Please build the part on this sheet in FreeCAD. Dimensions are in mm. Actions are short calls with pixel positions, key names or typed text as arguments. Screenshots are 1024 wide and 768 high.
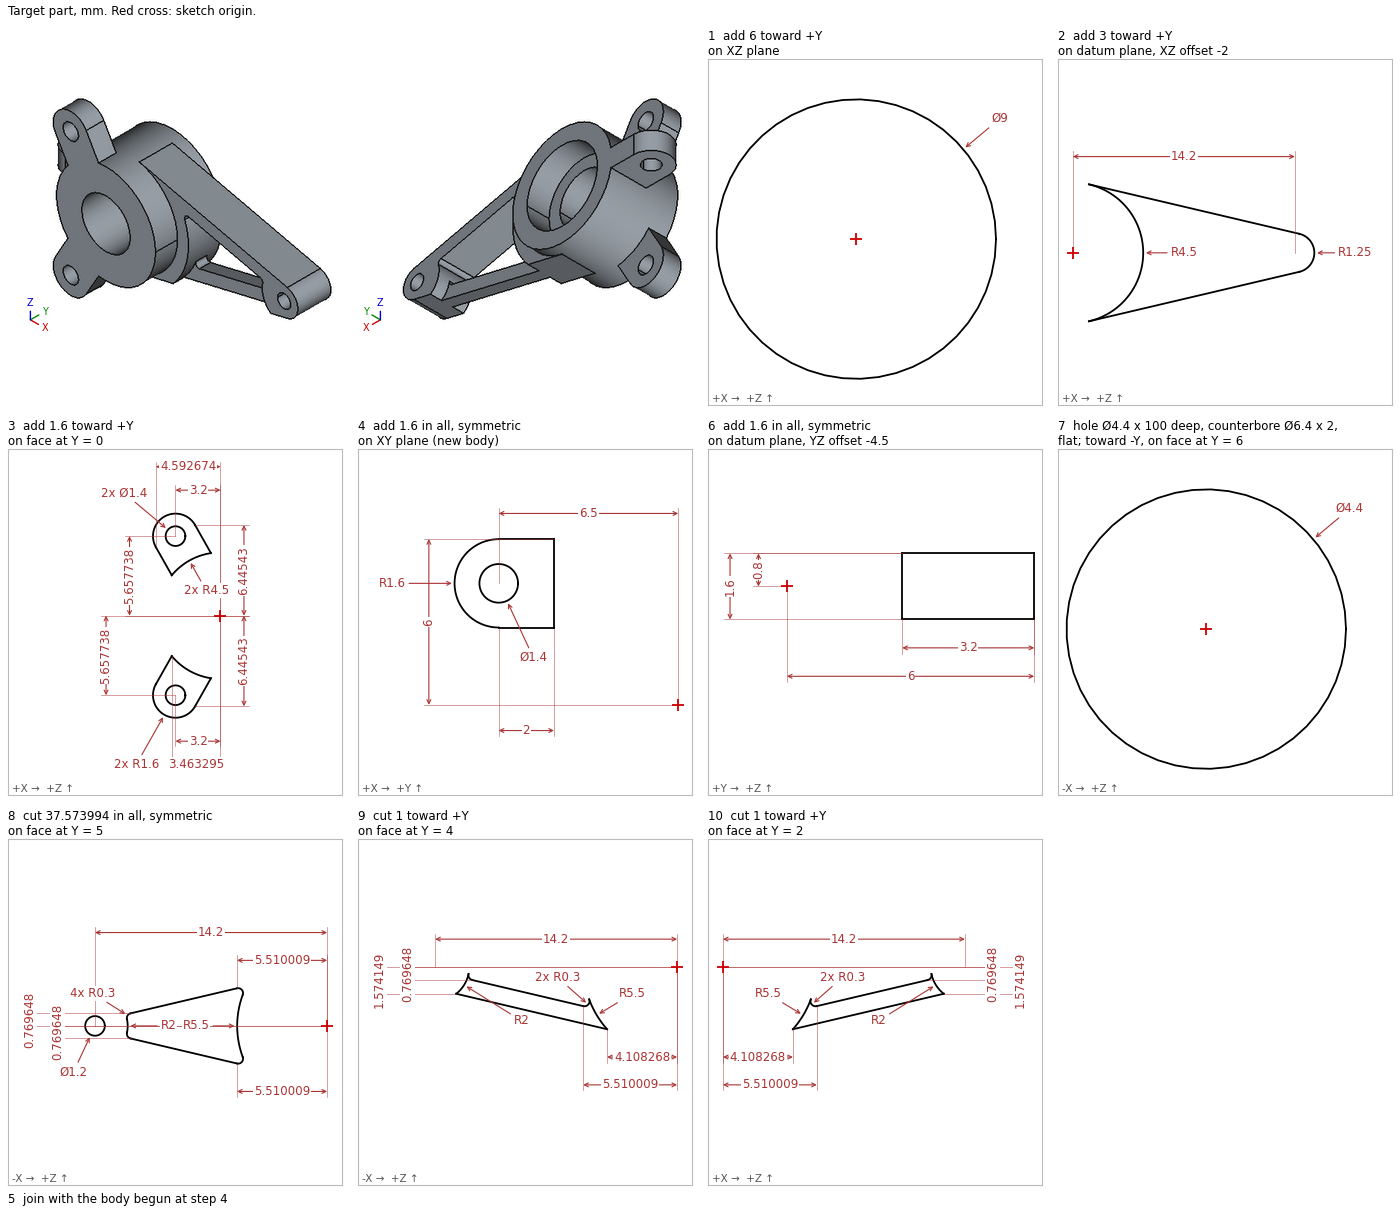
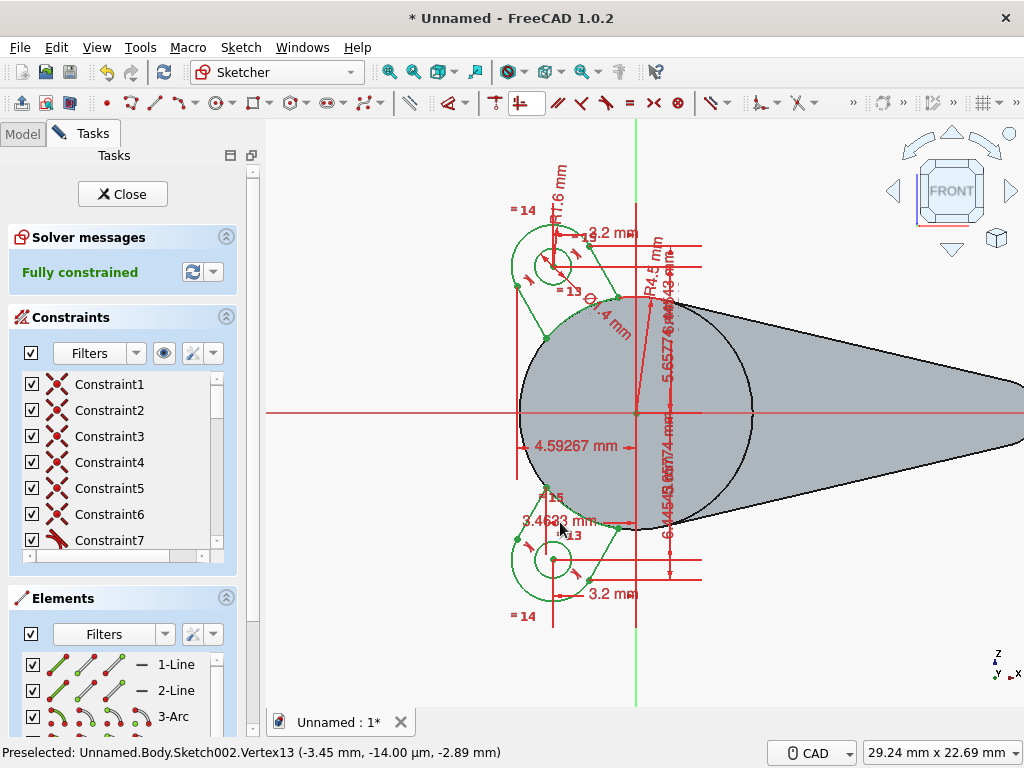
click(123, 194)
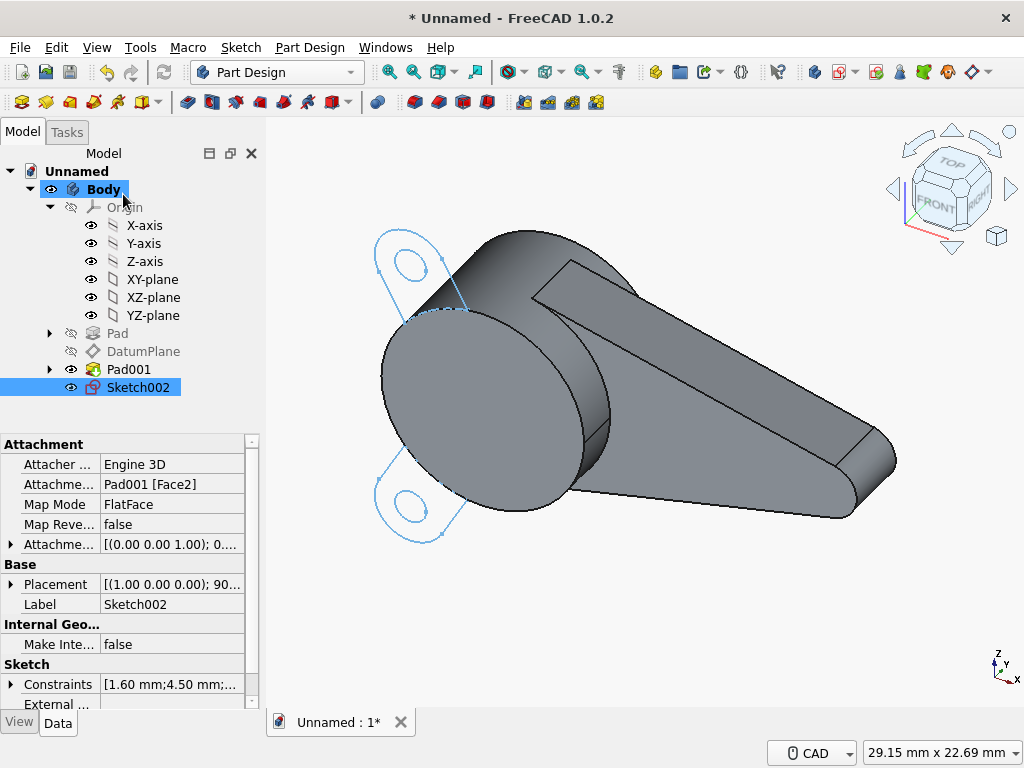
click(22, 102)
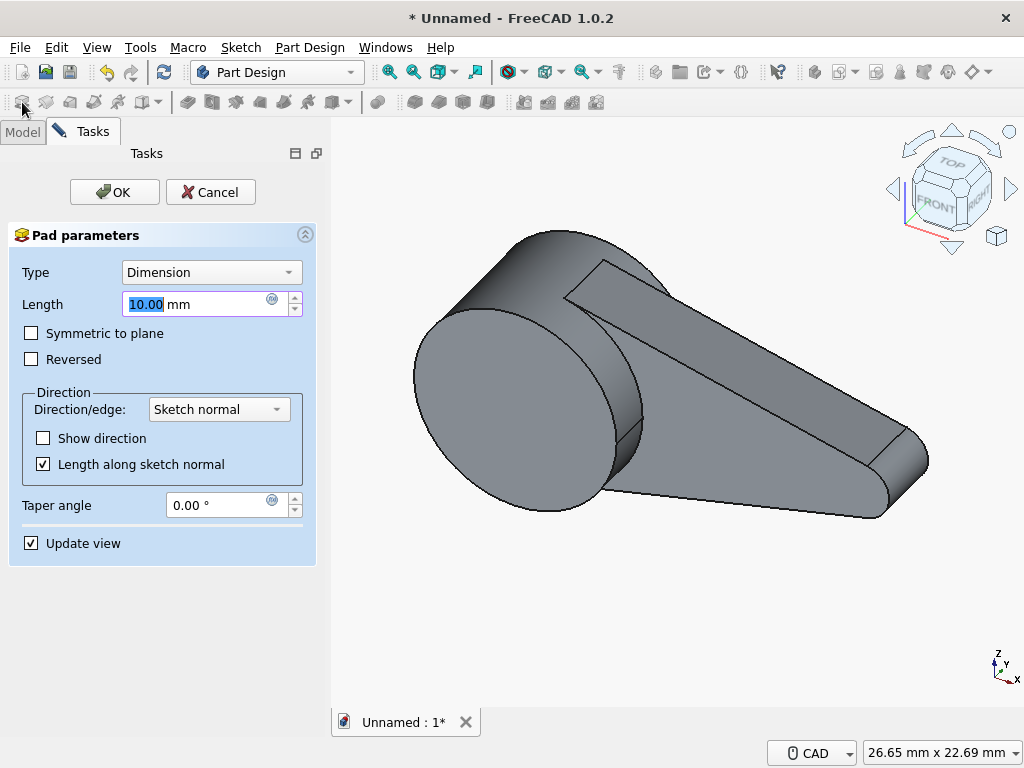
text(1.6)
key(Tab)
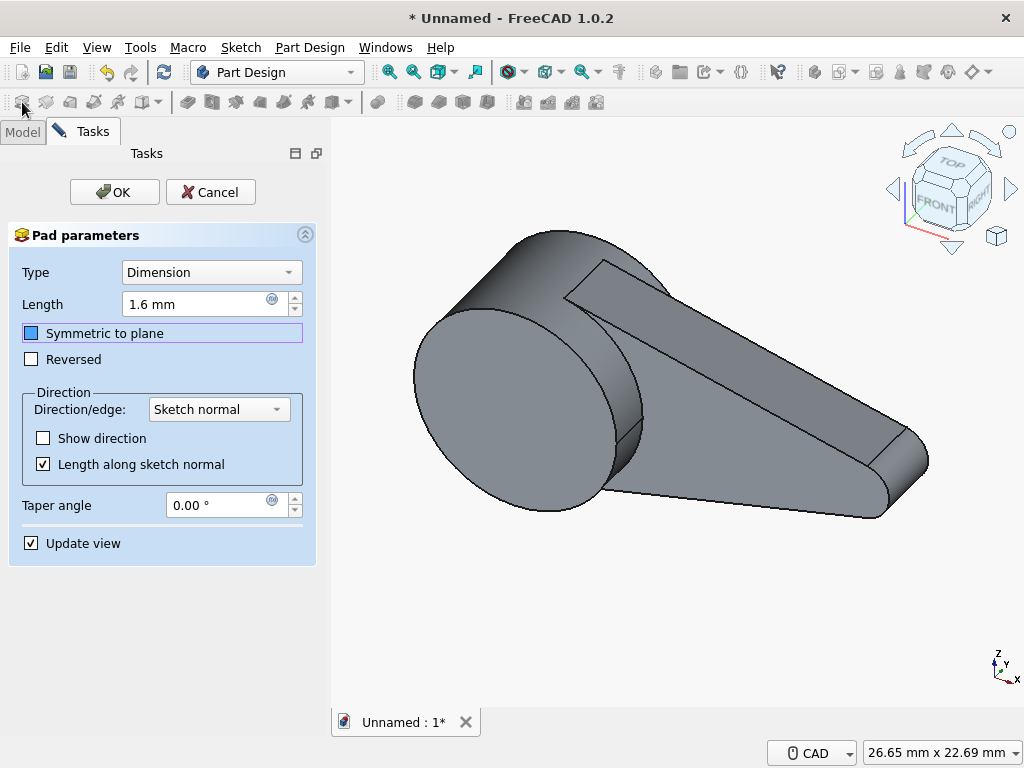
click(30, 359)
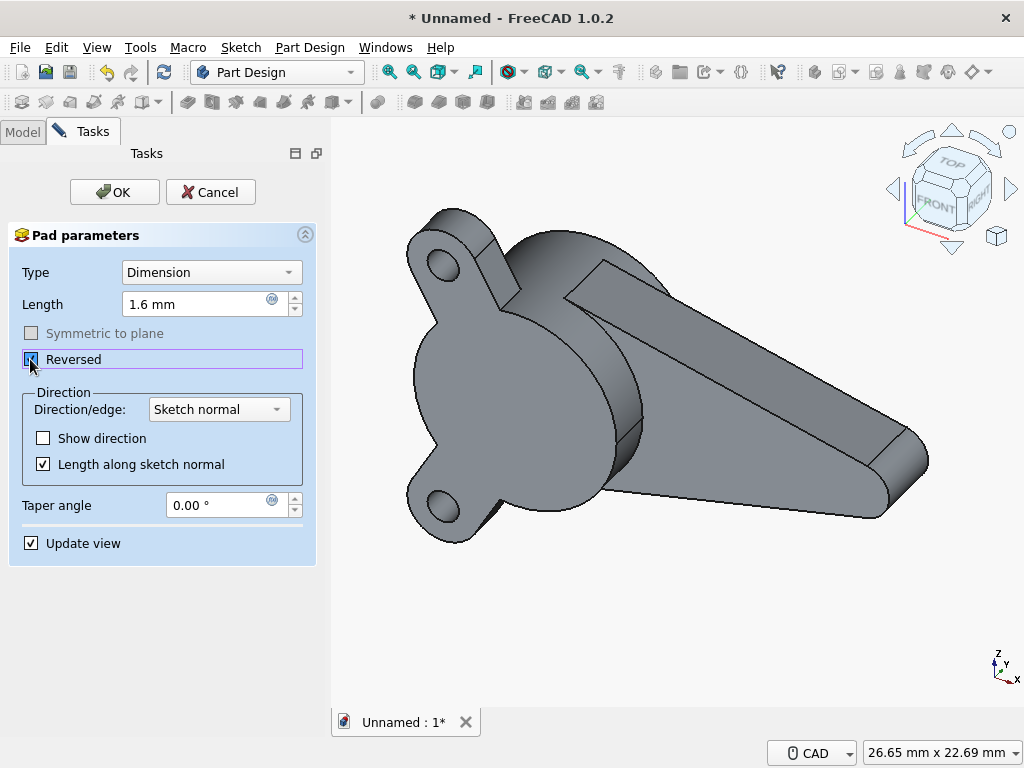
click(115, 192)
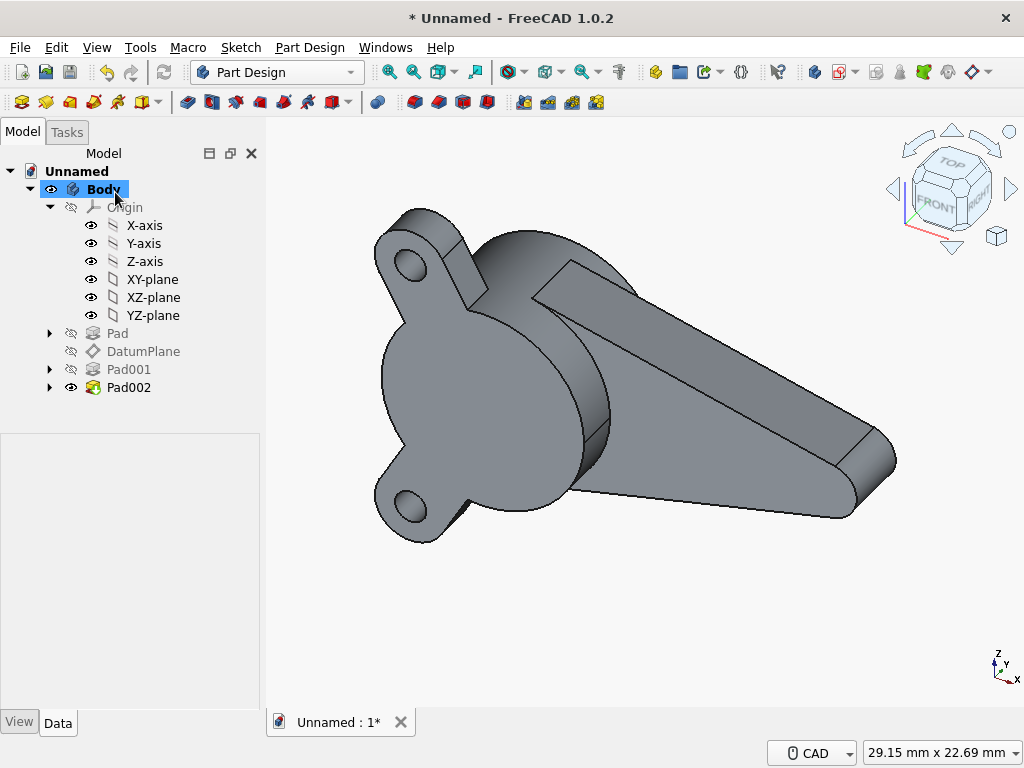
click(816, 72)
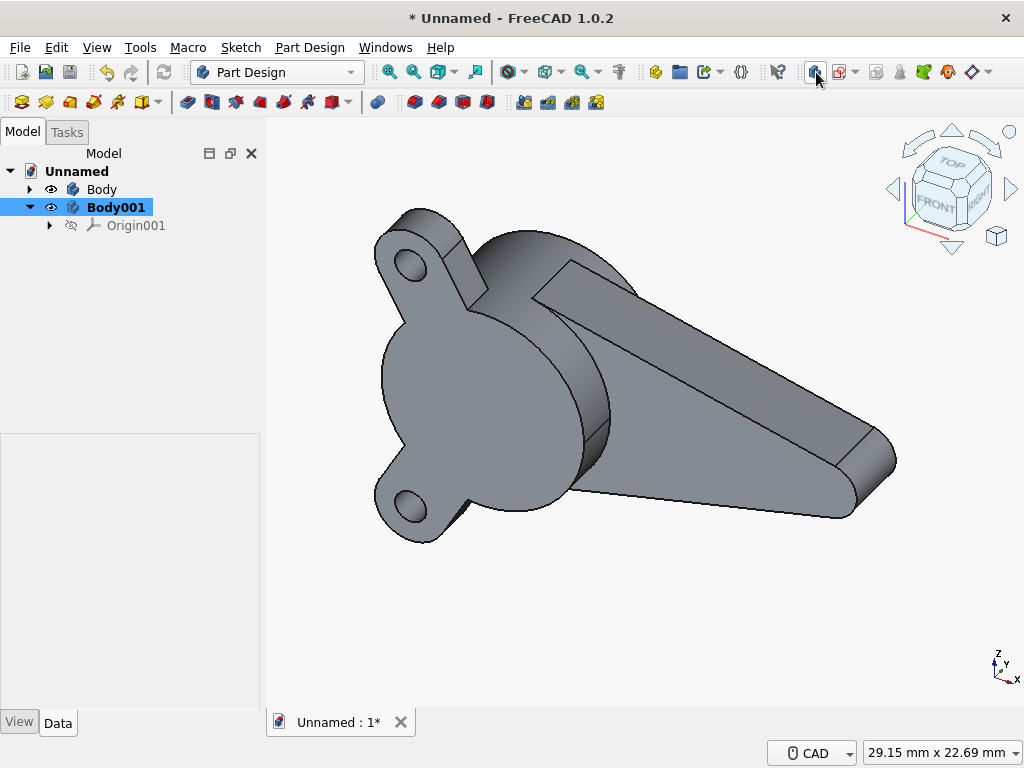
click(306, 667)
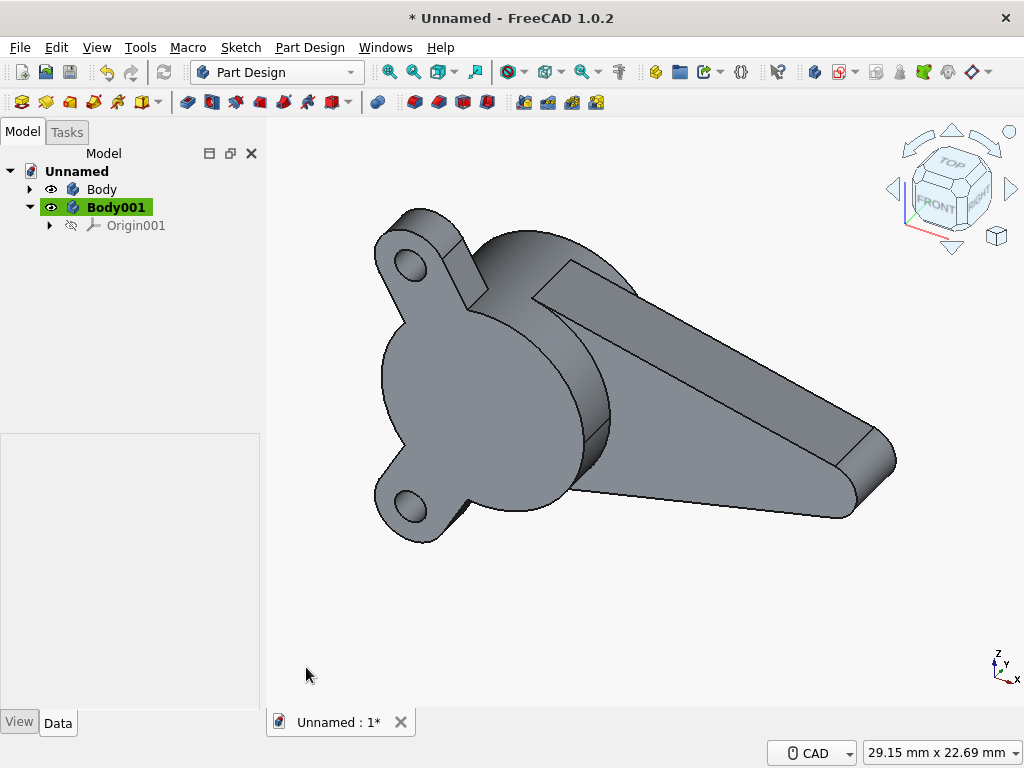
click(840, 72)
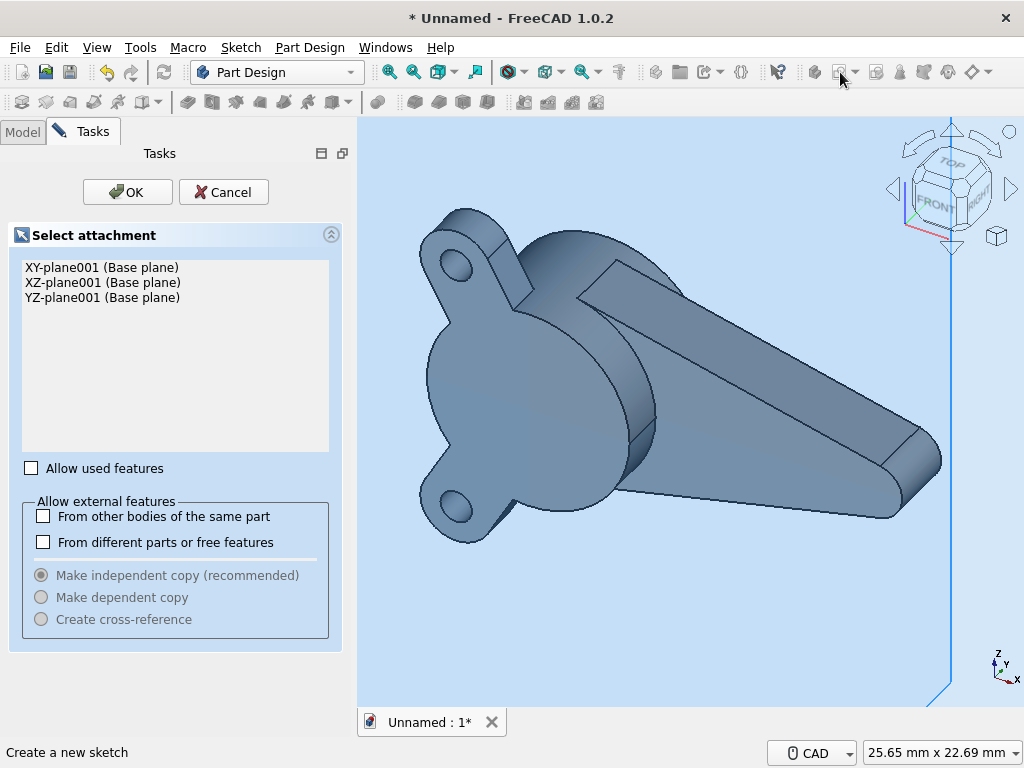
click(82, 268)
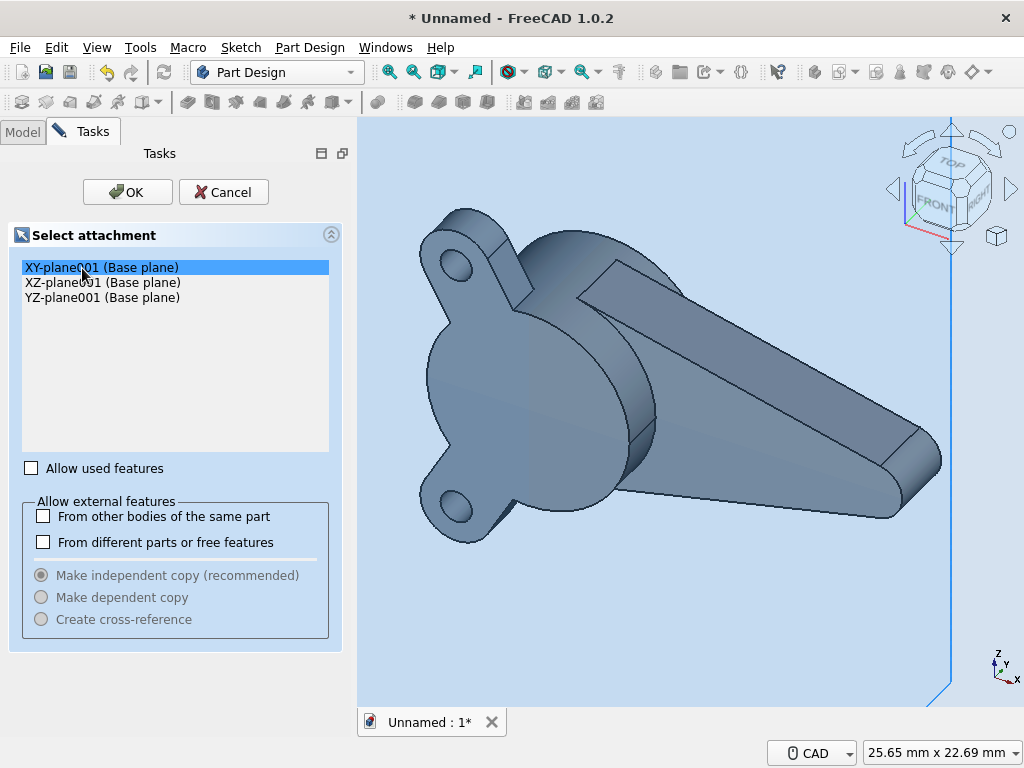
click(128, 192)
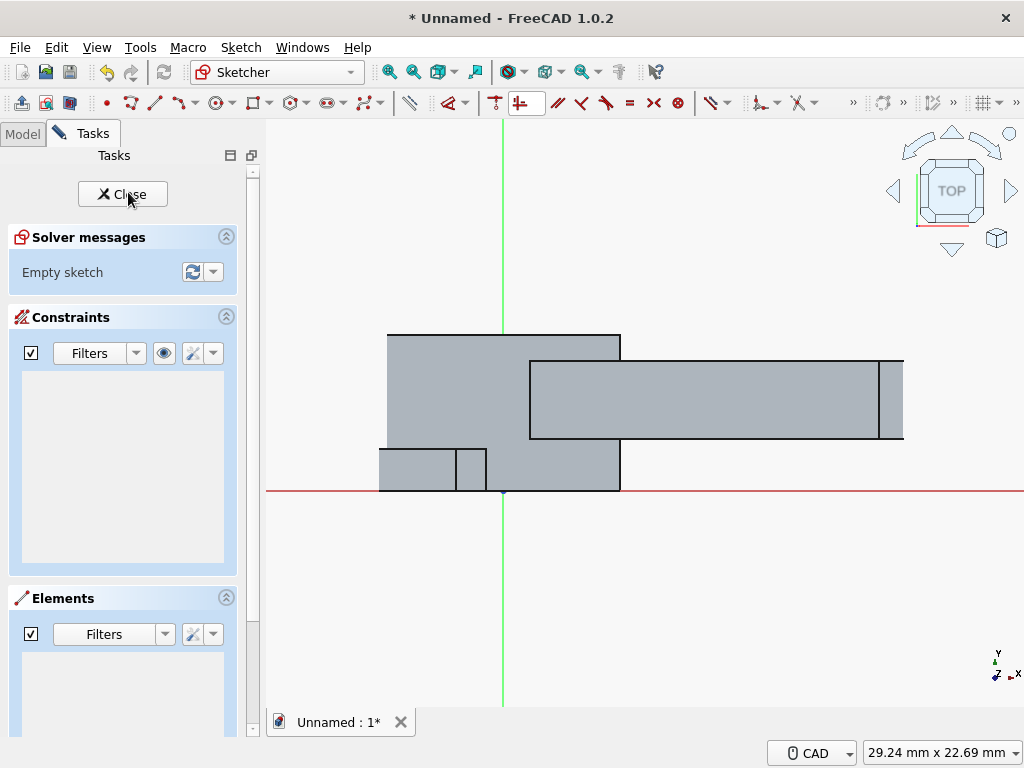
scroll(576, 413, down, 5)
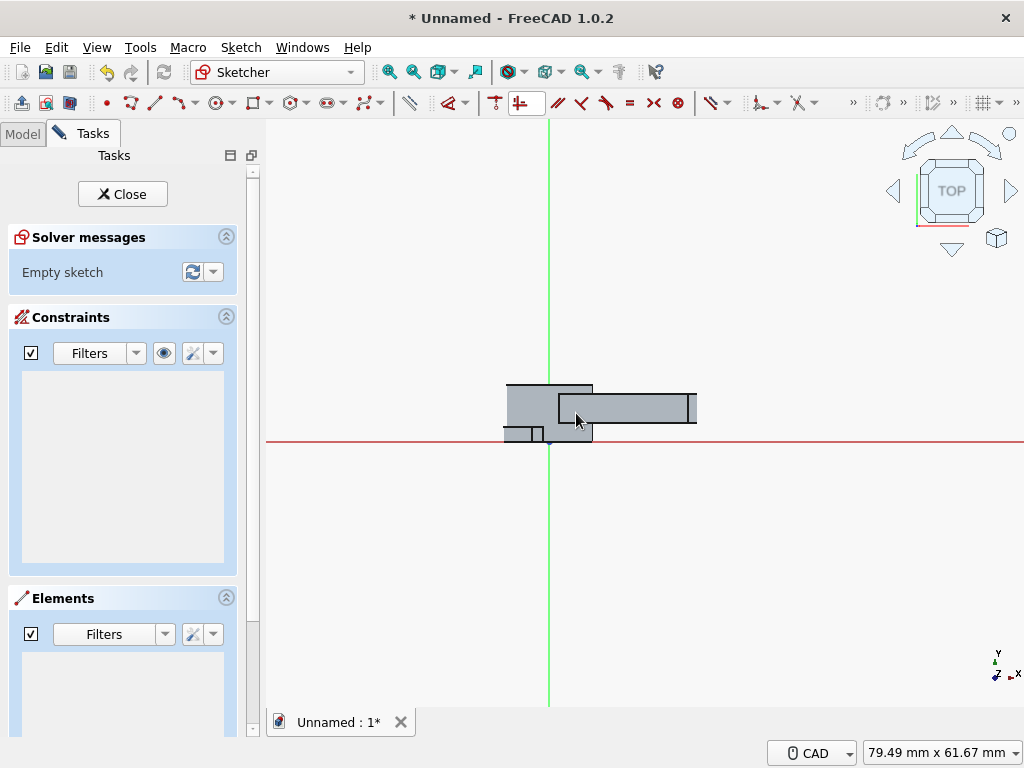
scroll(494, 413, up, 8)